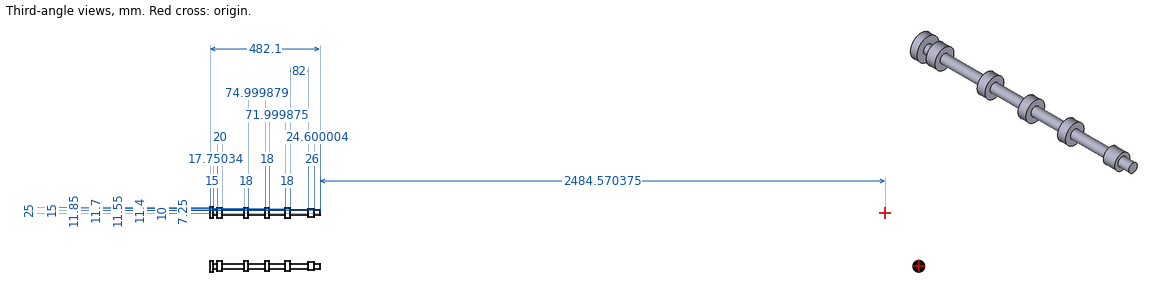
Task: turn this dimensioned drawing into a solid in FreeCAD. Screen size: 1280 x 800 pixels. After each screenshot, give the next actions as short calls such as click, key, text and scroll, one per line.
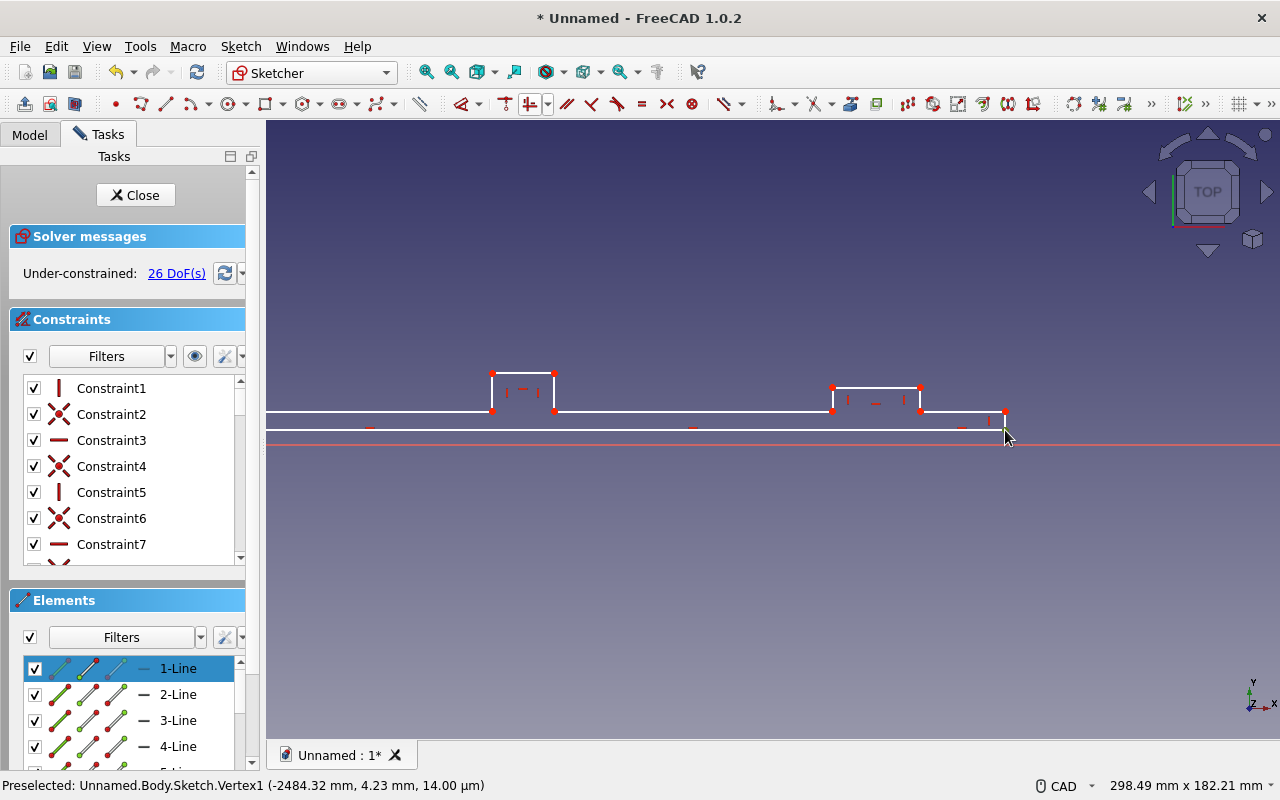
click(1056, 445)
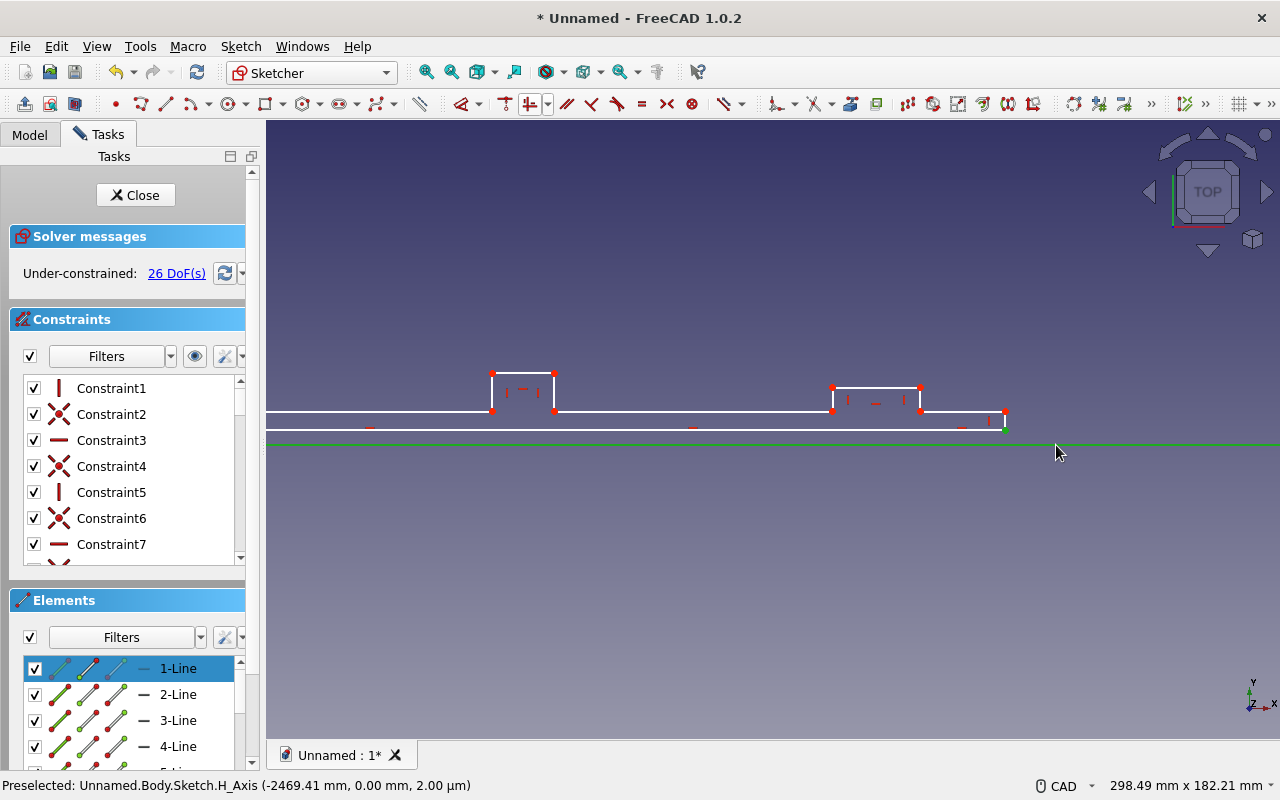
click(505, 104)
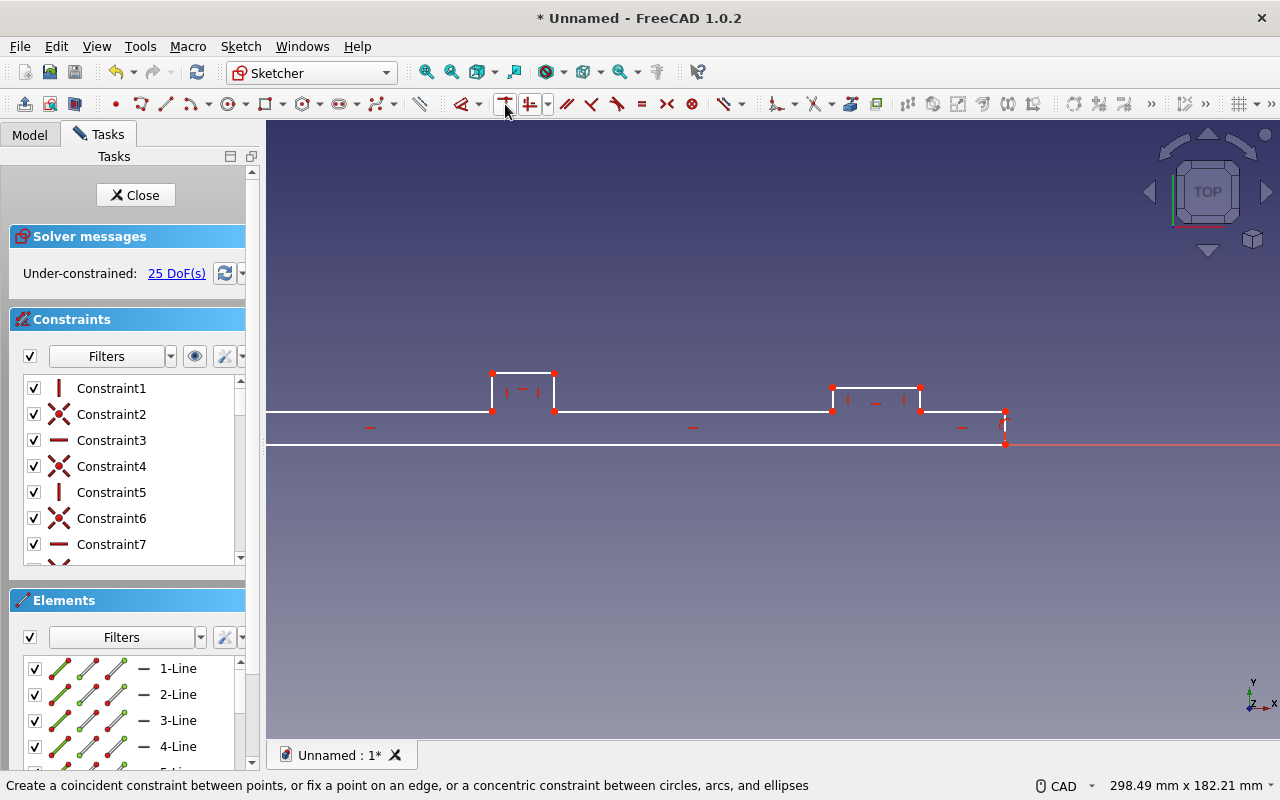
scroll(1005, 435, up, 2)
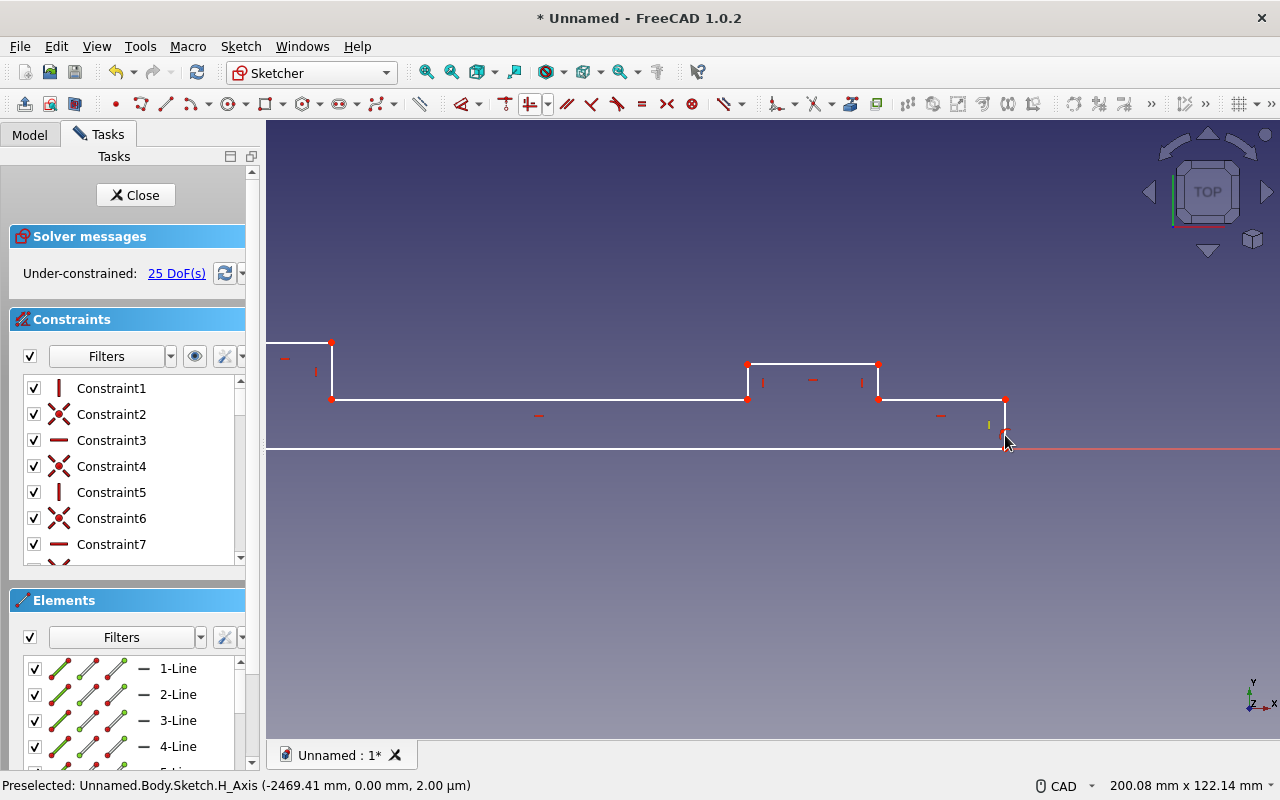
click(1005, 415)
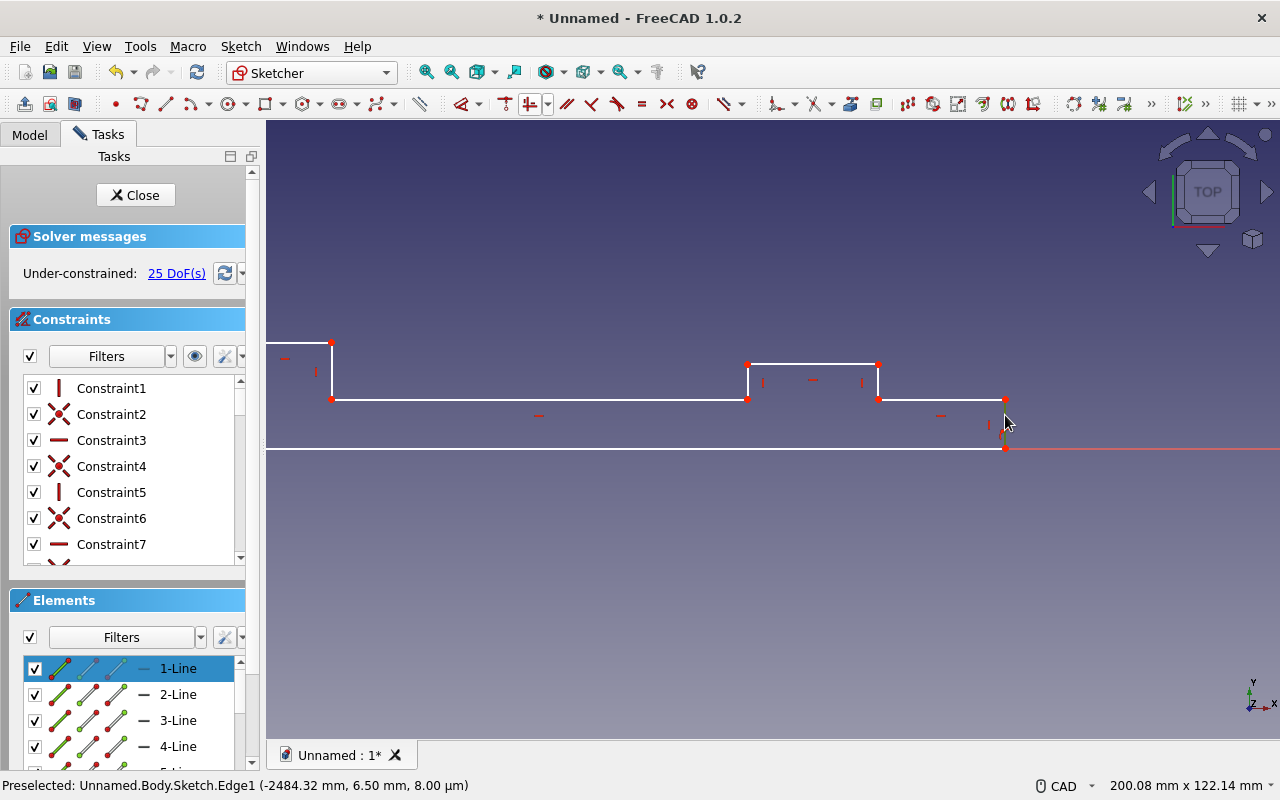
key(i)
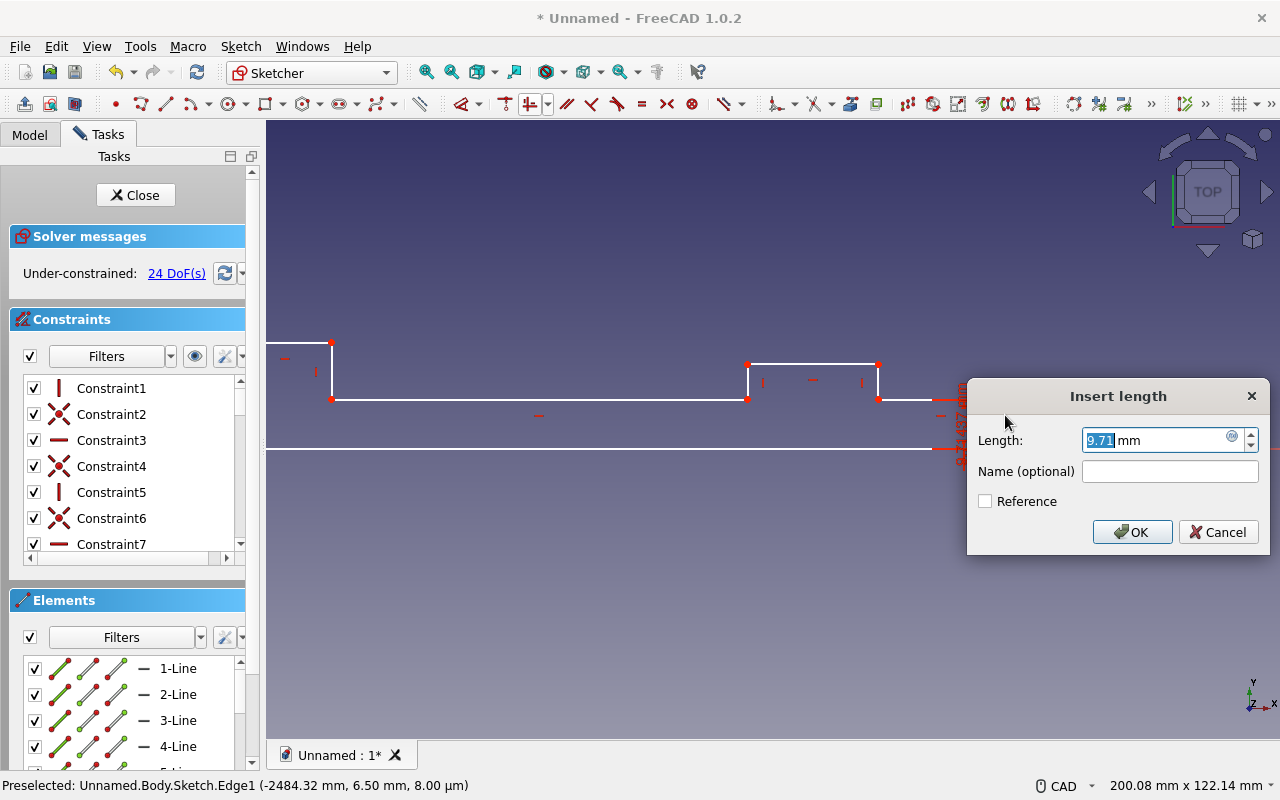
text(10)
key(Return)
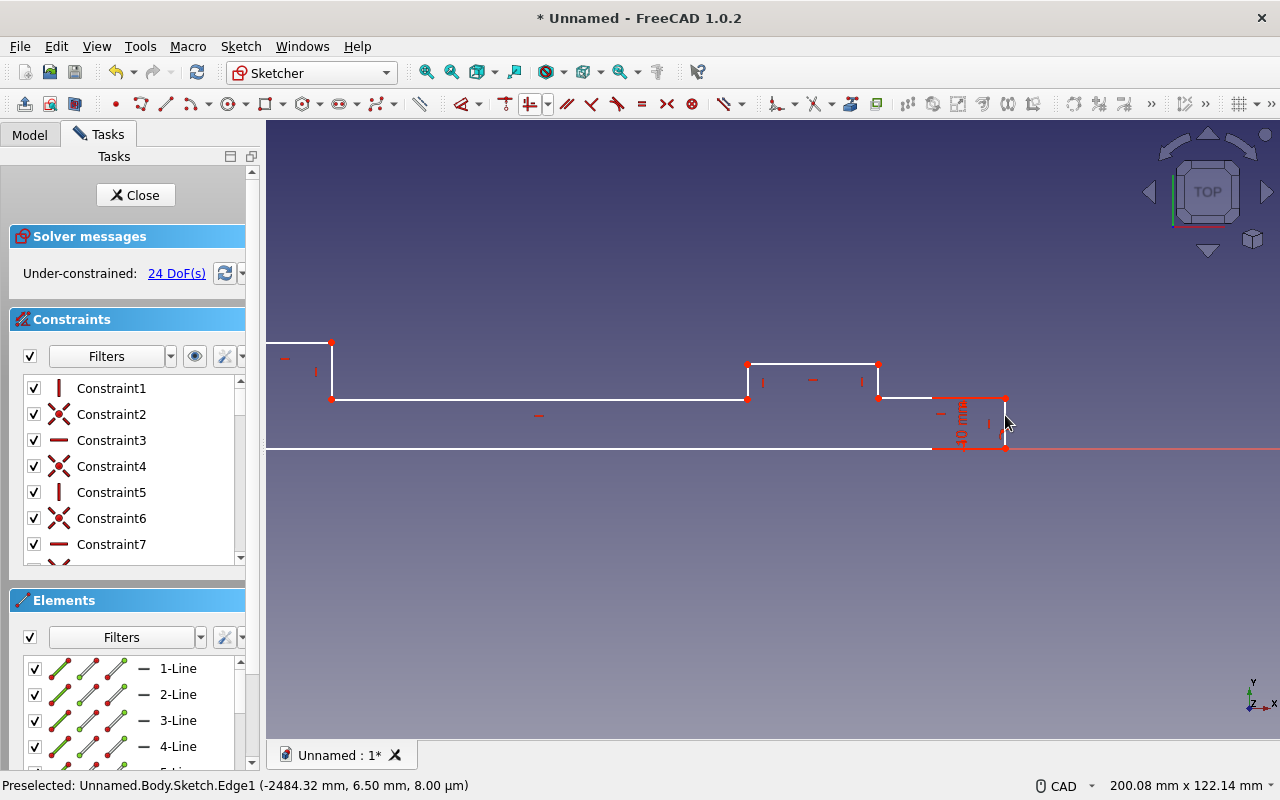
click(839, 364)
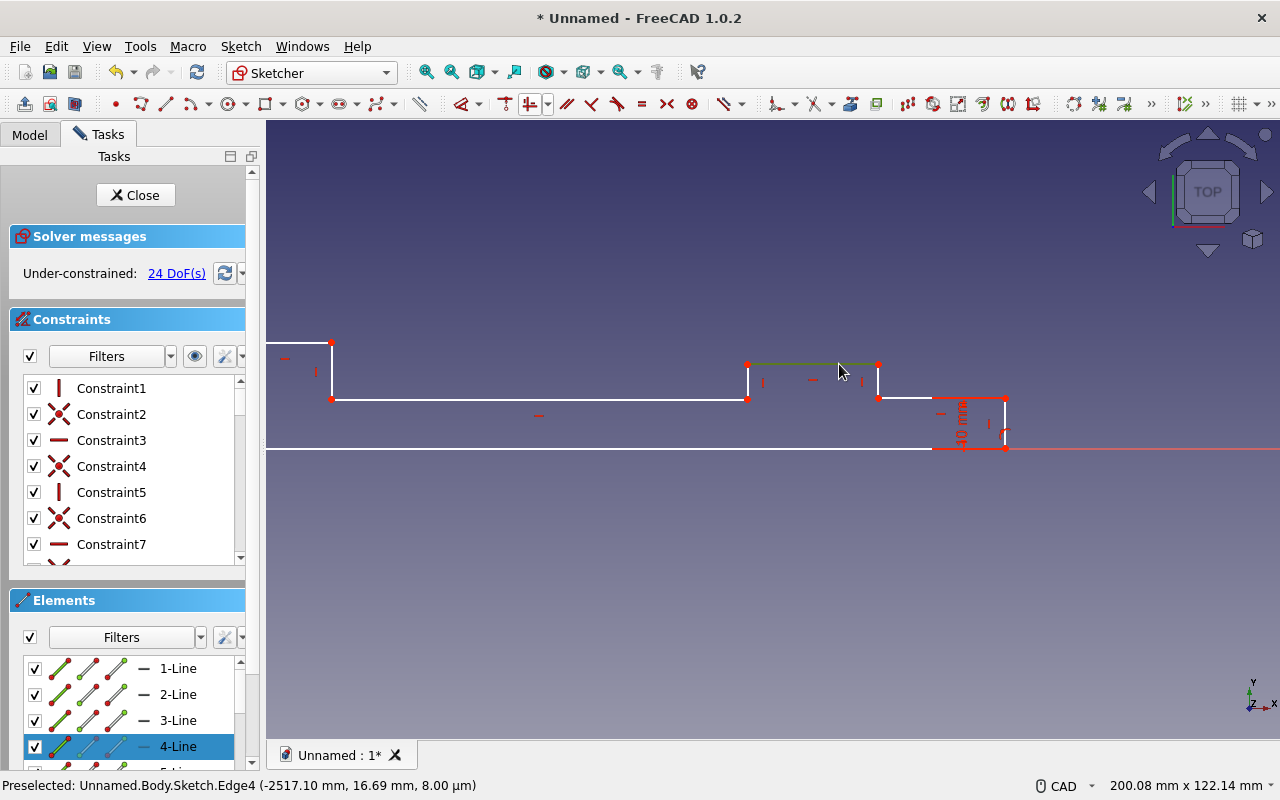
click(478, 104)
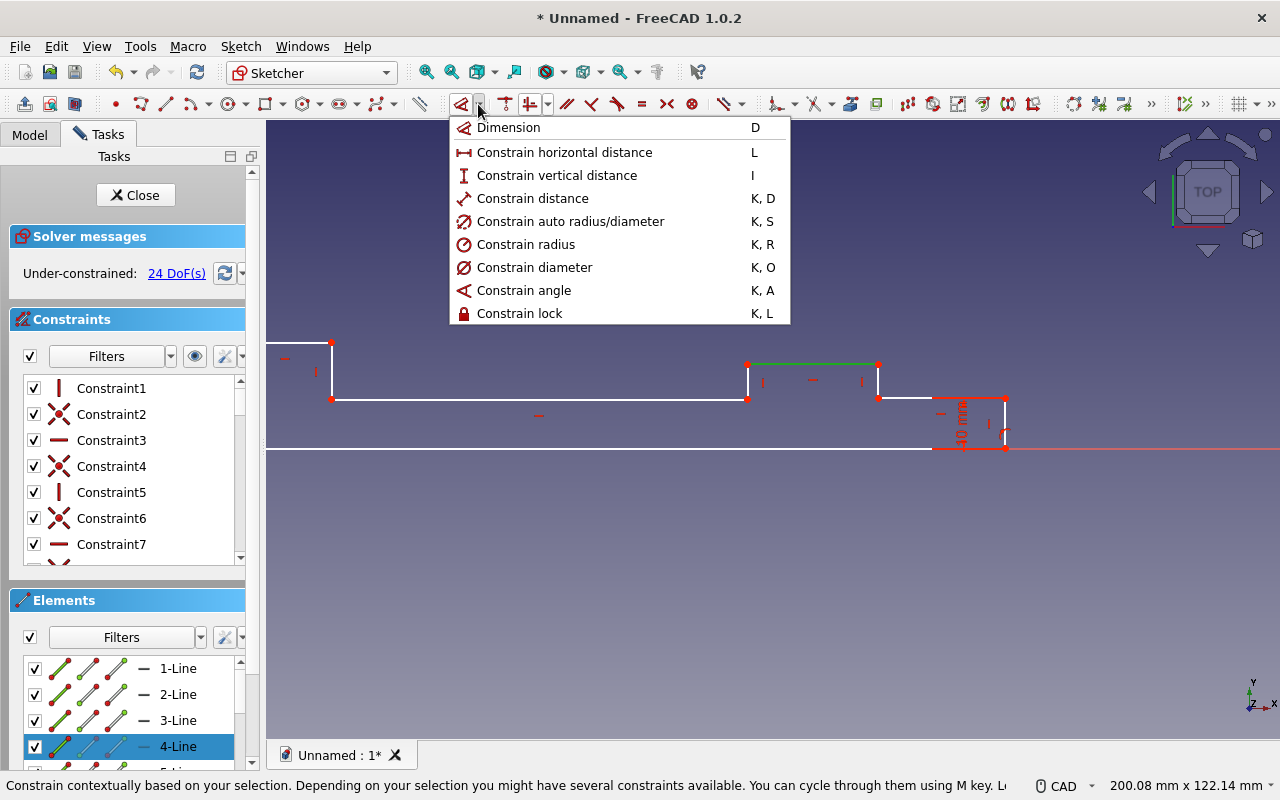
click(620, 152)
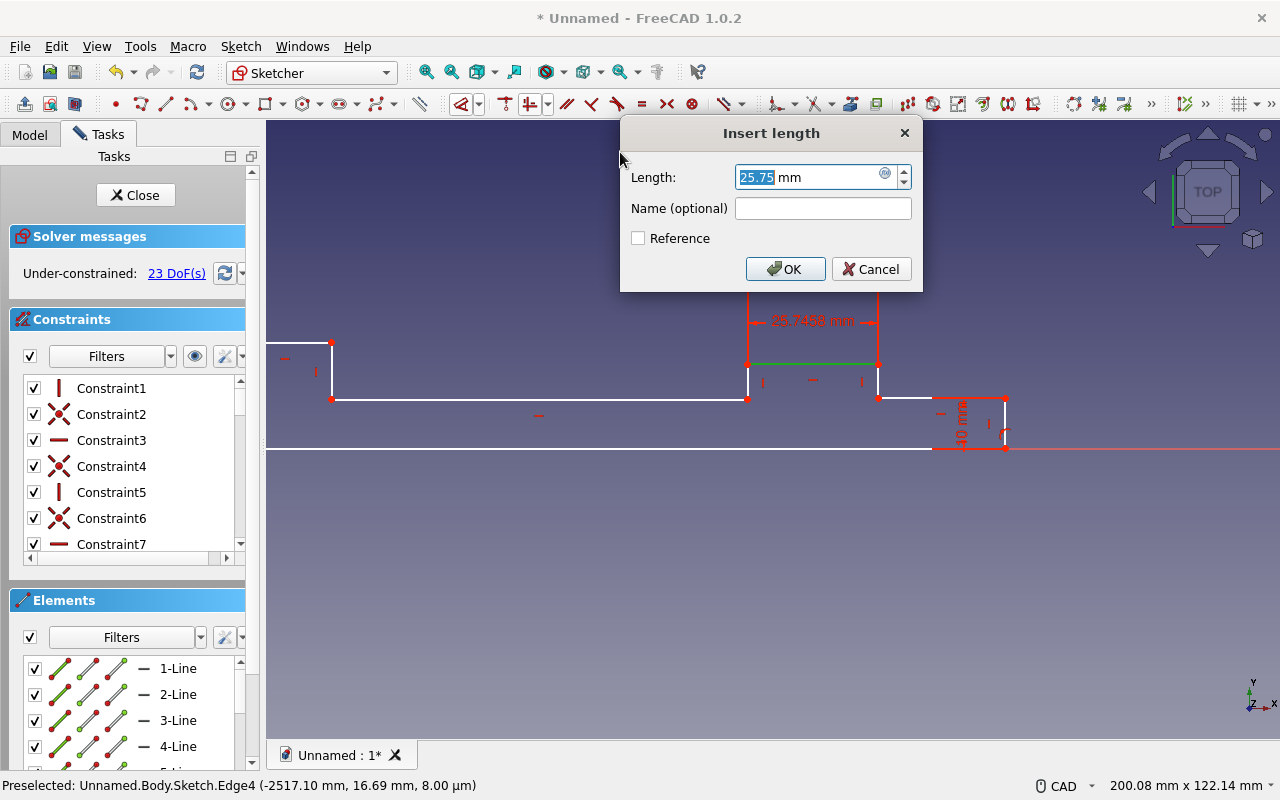
text(26)
key(Return)